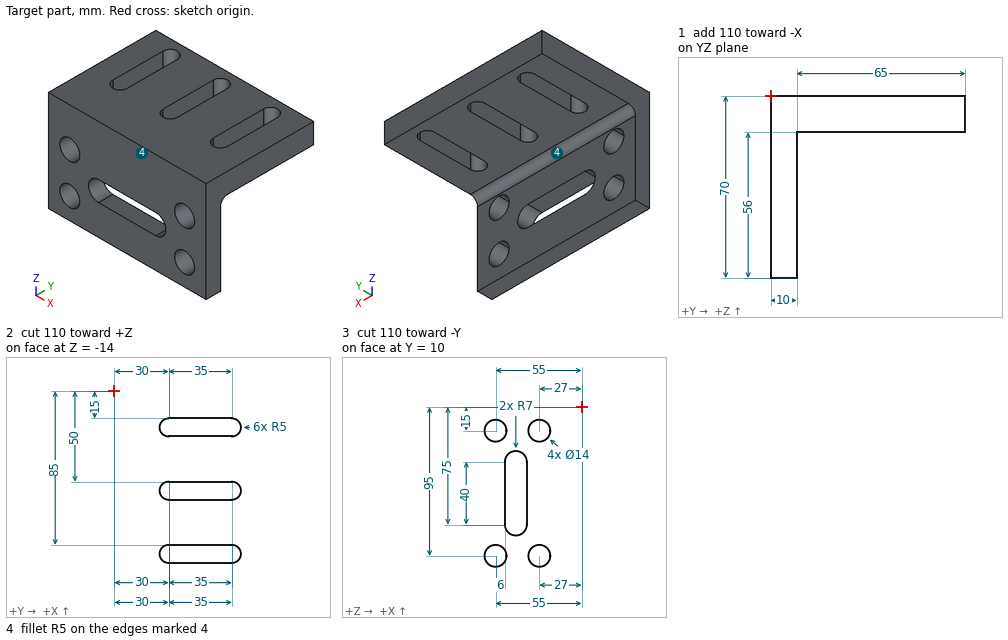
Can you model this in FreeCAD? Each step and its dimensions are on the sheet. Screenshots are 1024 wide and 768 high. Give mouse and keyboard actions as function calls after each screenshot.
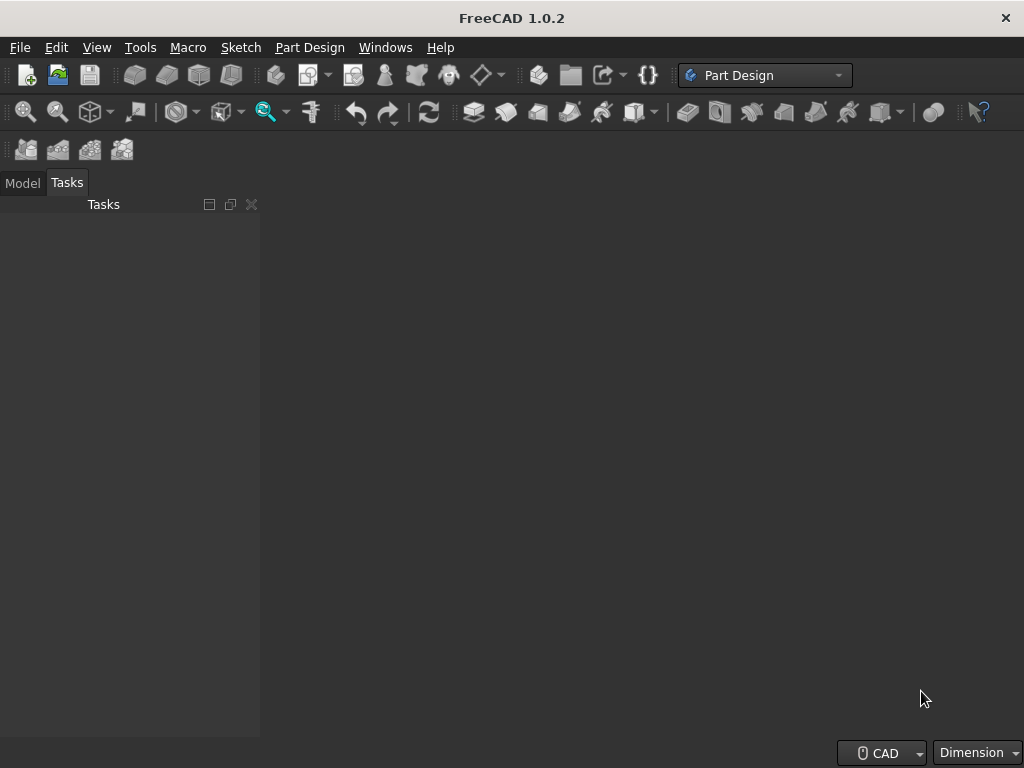
key(ctrl+n)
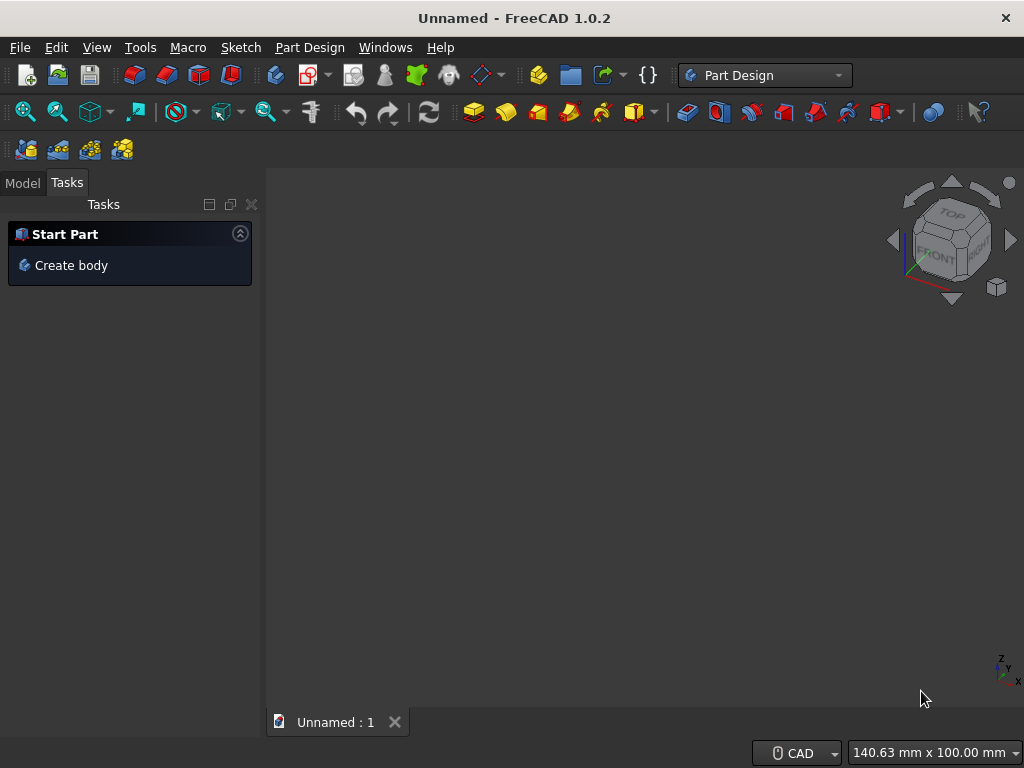
click(308, 76)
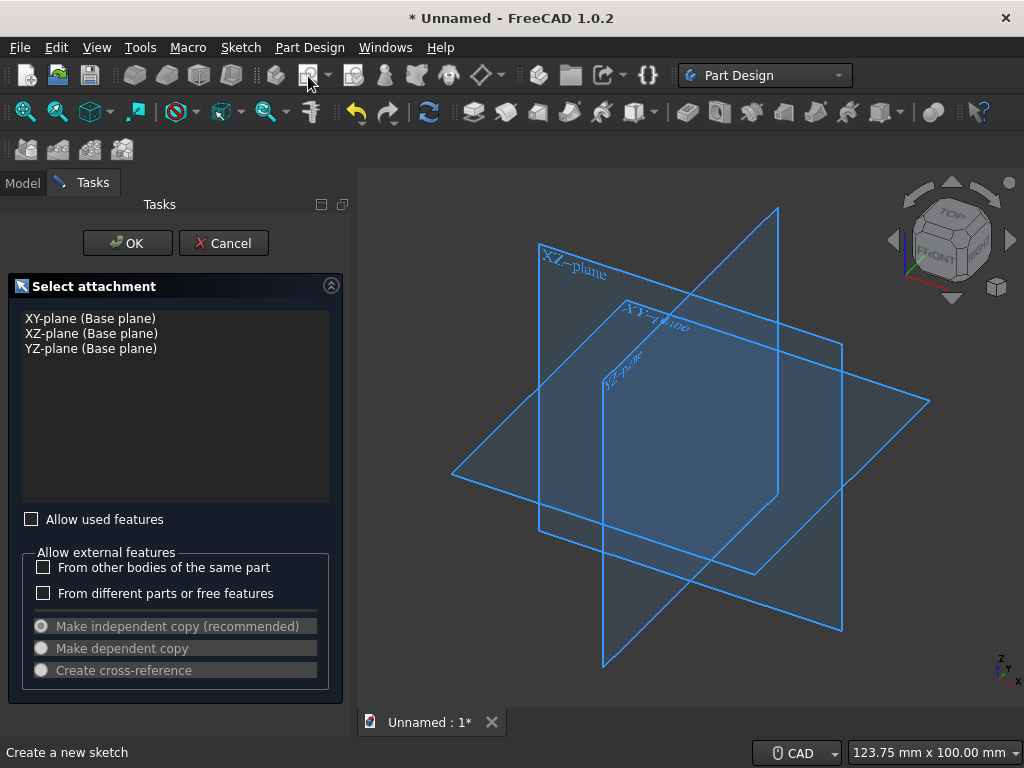
click(82, 348)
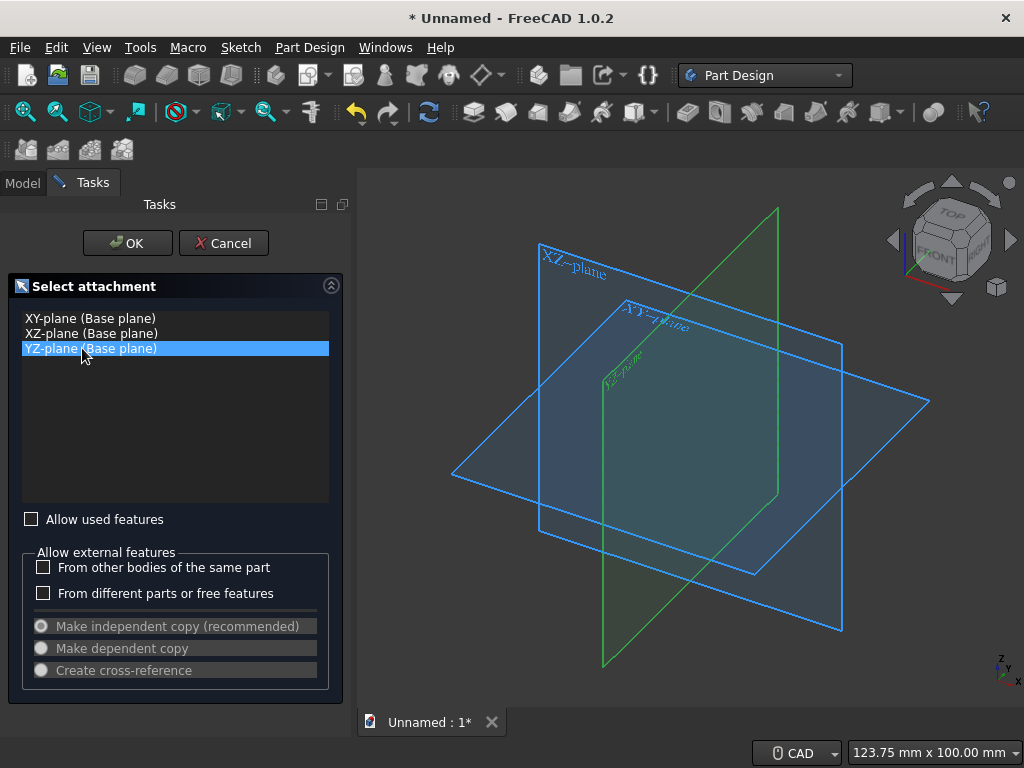
click(128, 243)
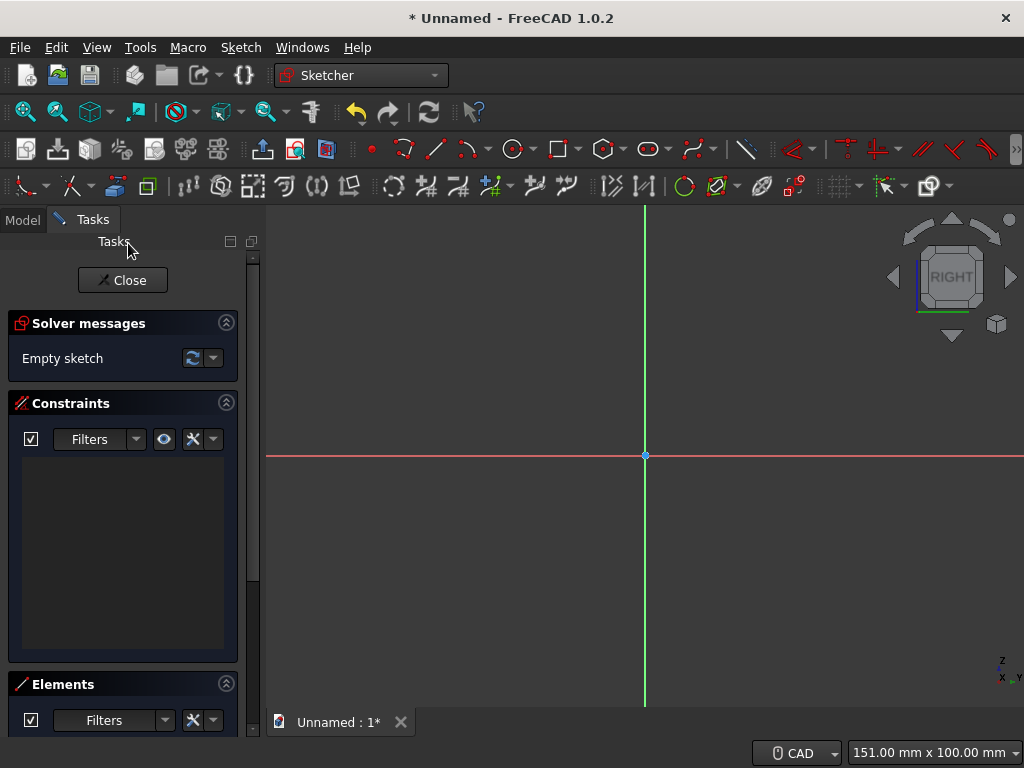
scroll(294, 233, down, 2)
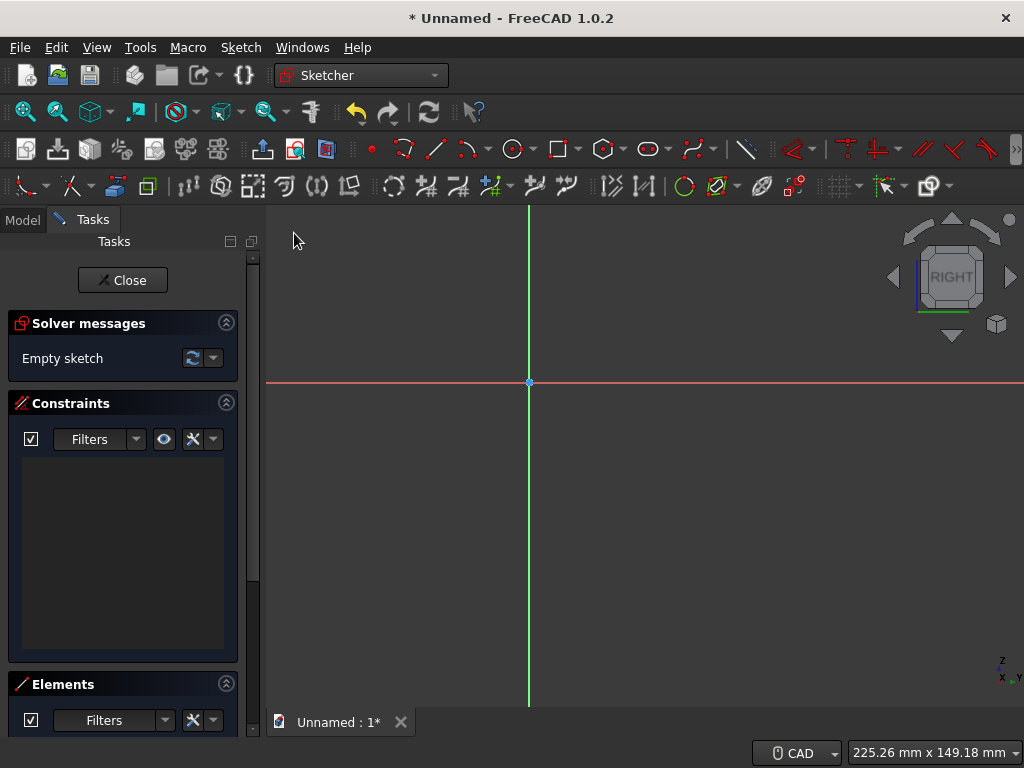
key(g)
key(m)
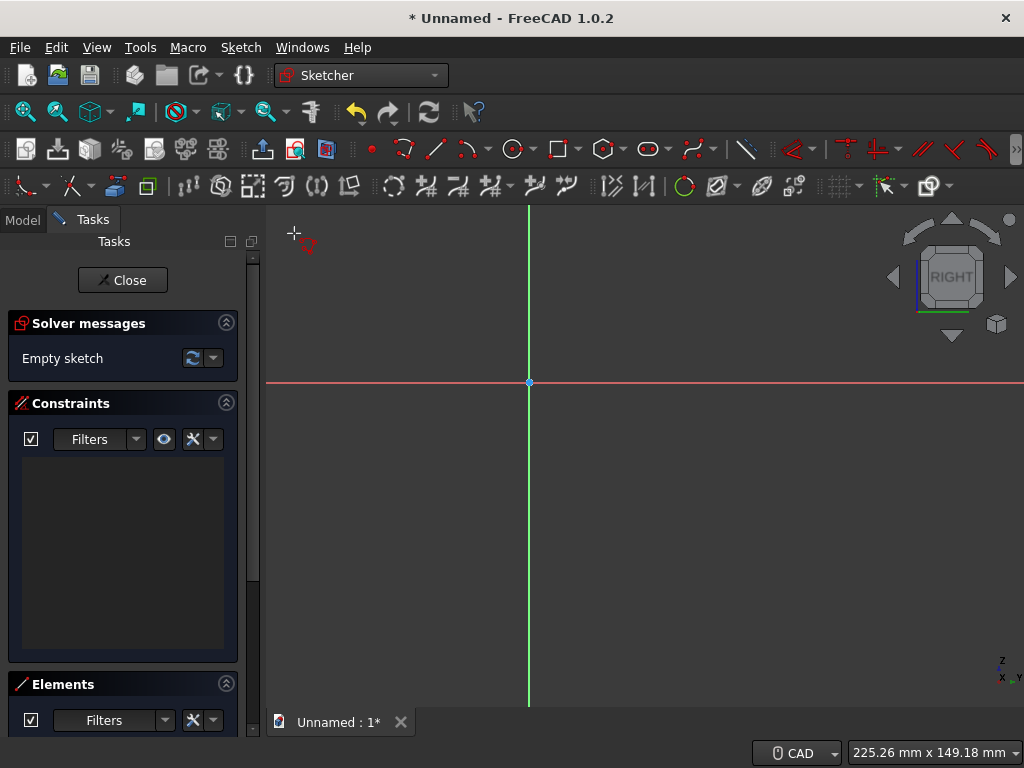
click(529, 382)
click(538, 618)
click(563, 618)
click(563, 430)
click(782, 430)
click(782, 391)
click(529, 382)
key(Escape)
key(Escape)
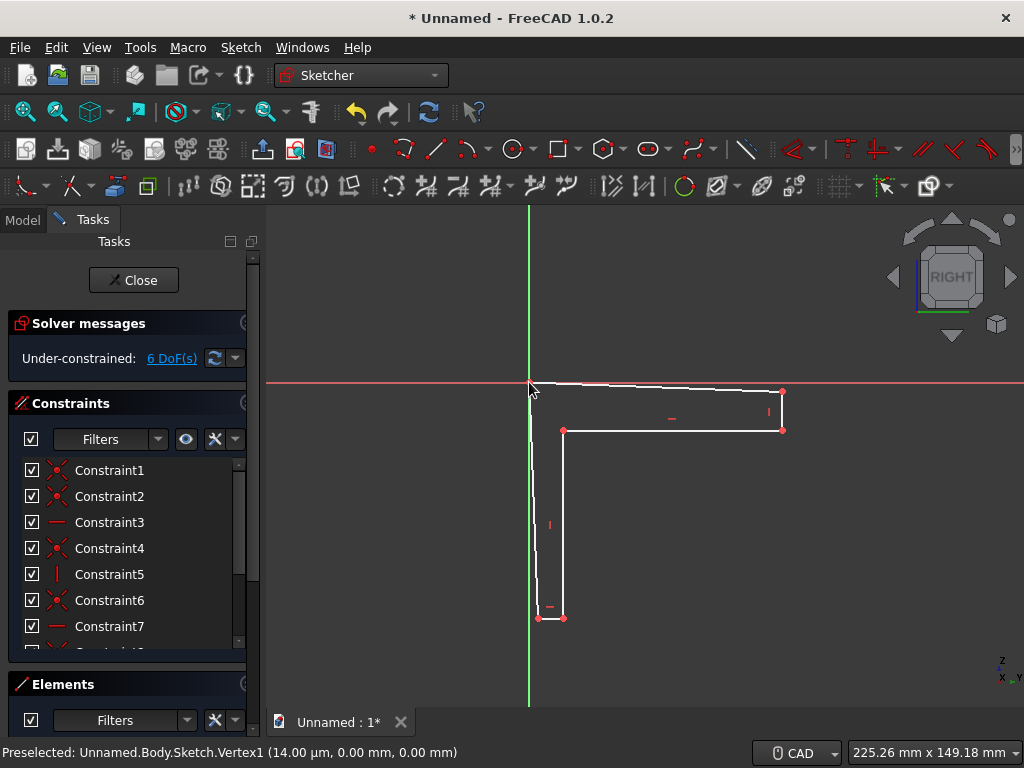
click(532, 453)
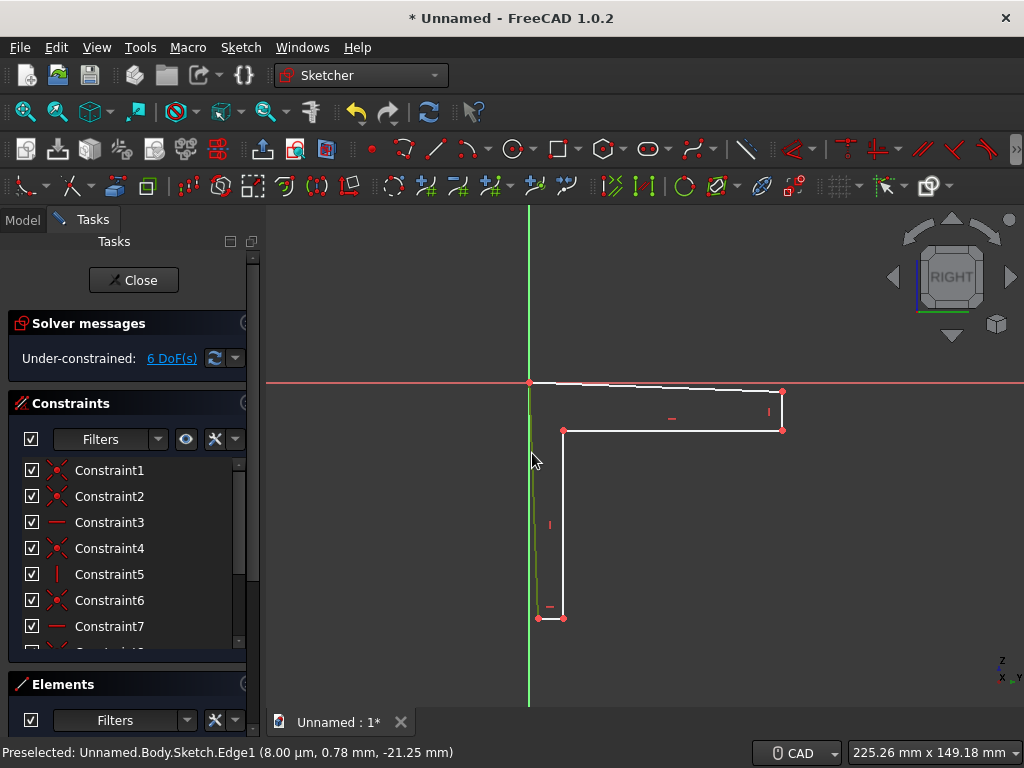
key(v)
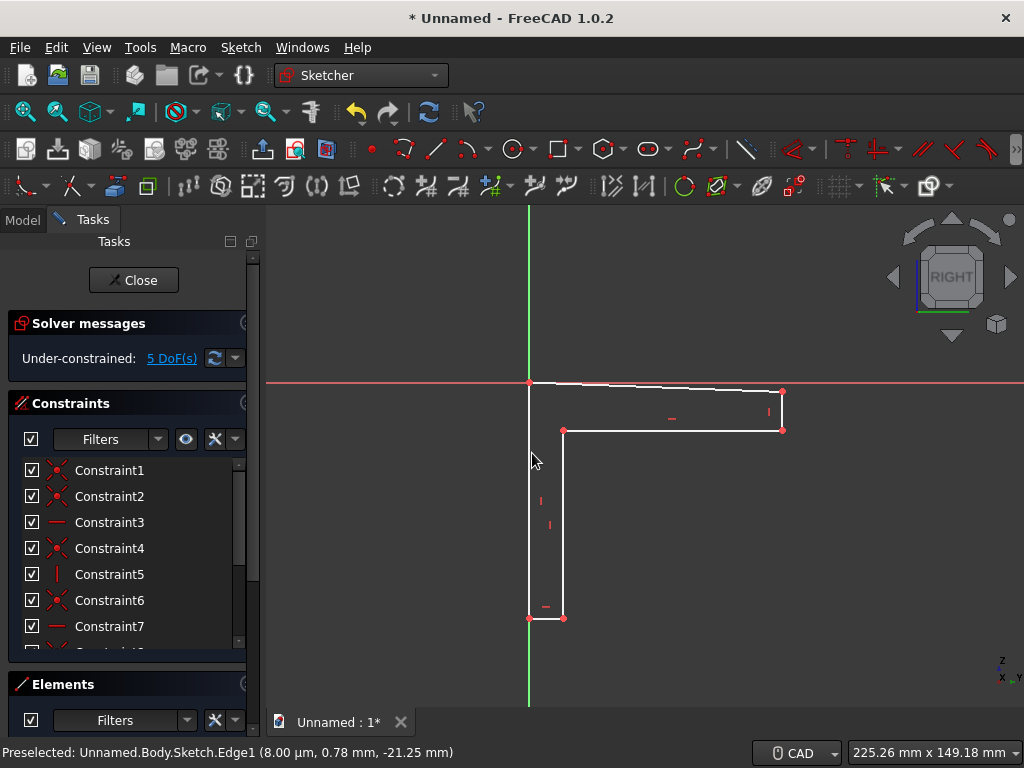
click(605, 385)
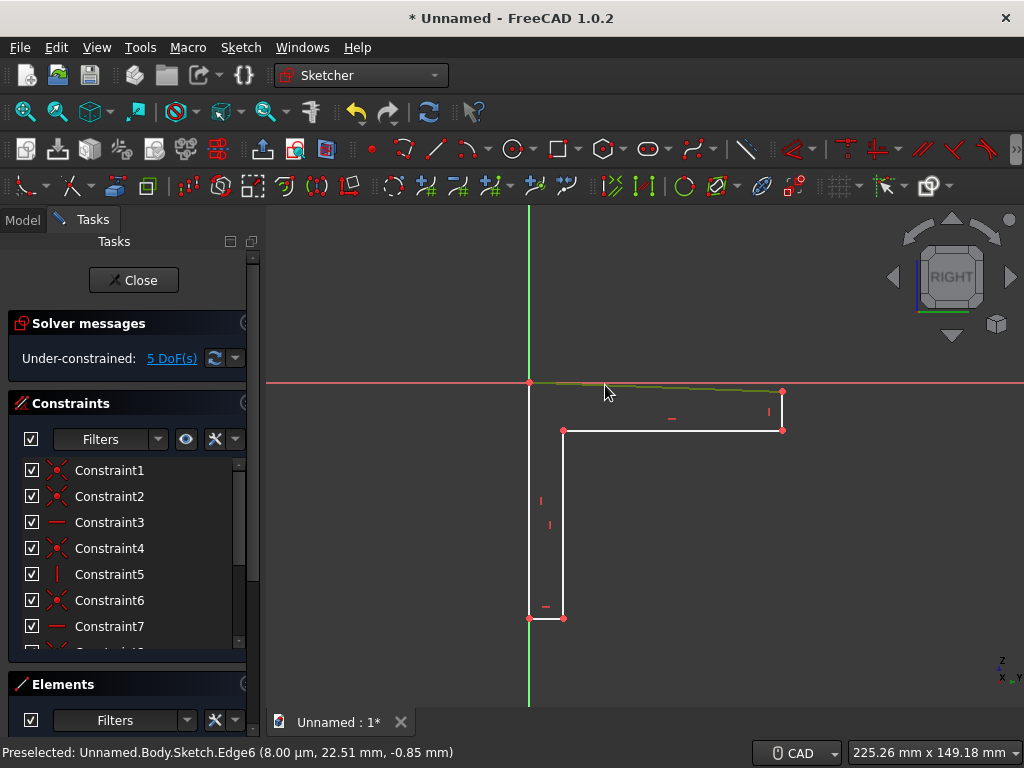
key(h)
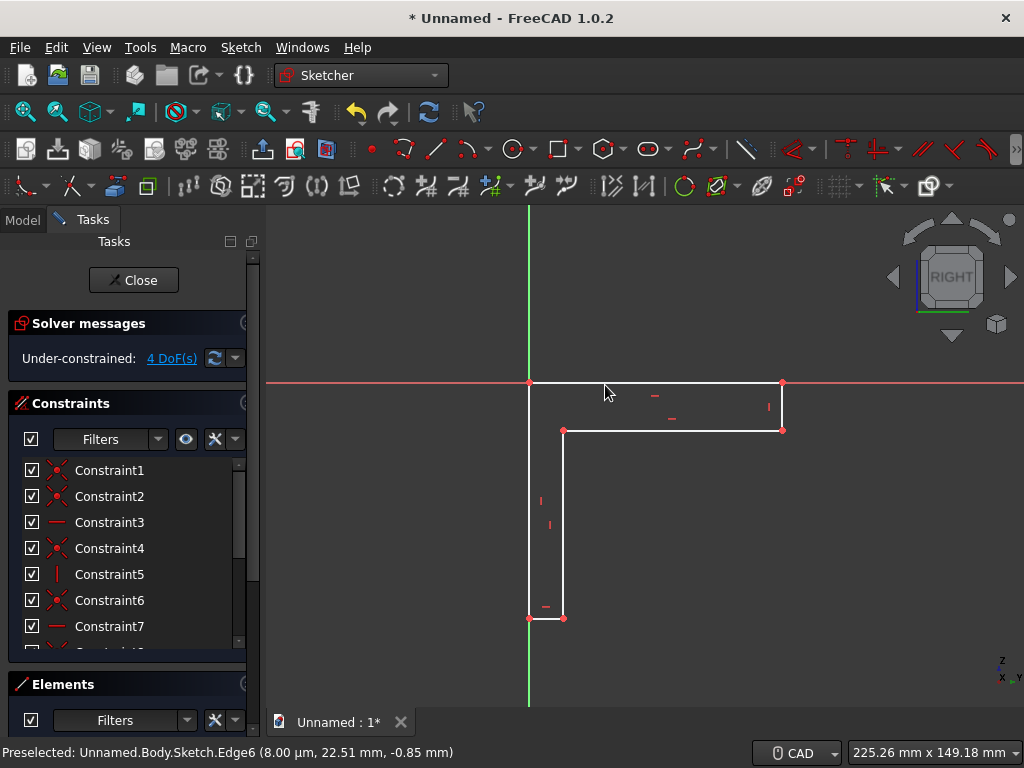
click(529, 453)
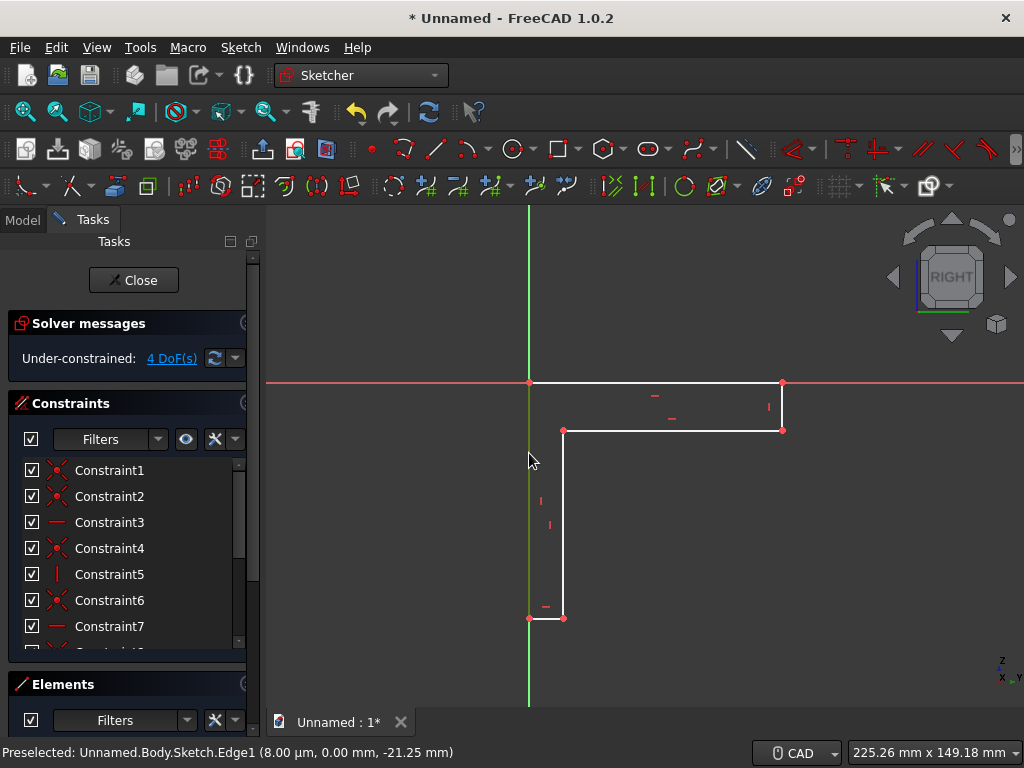
key(i)